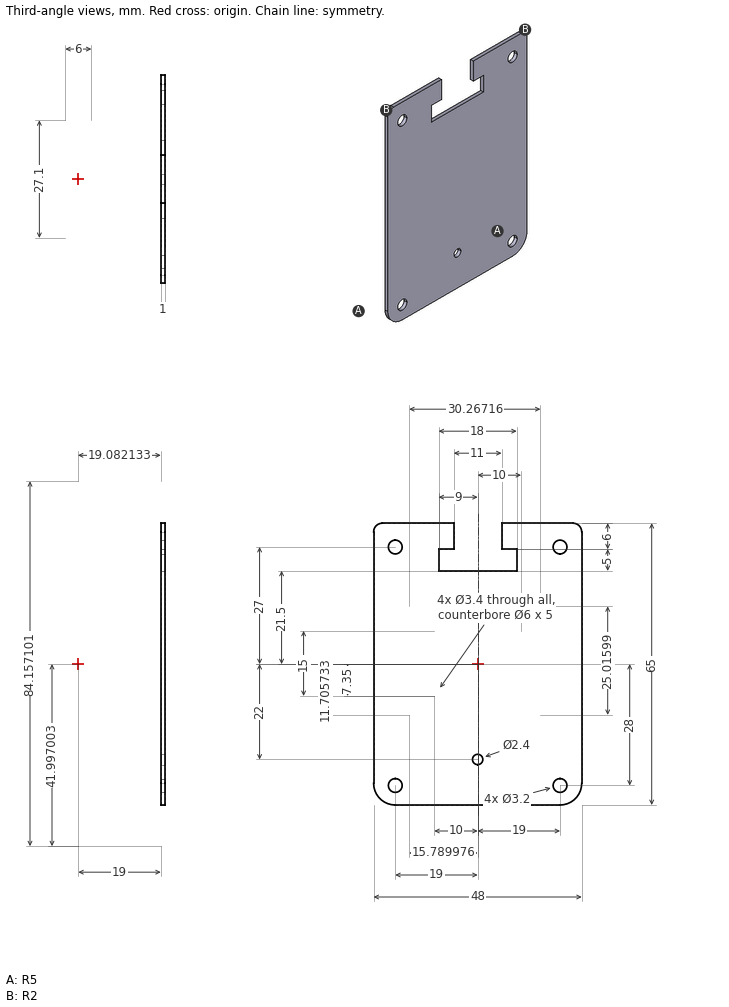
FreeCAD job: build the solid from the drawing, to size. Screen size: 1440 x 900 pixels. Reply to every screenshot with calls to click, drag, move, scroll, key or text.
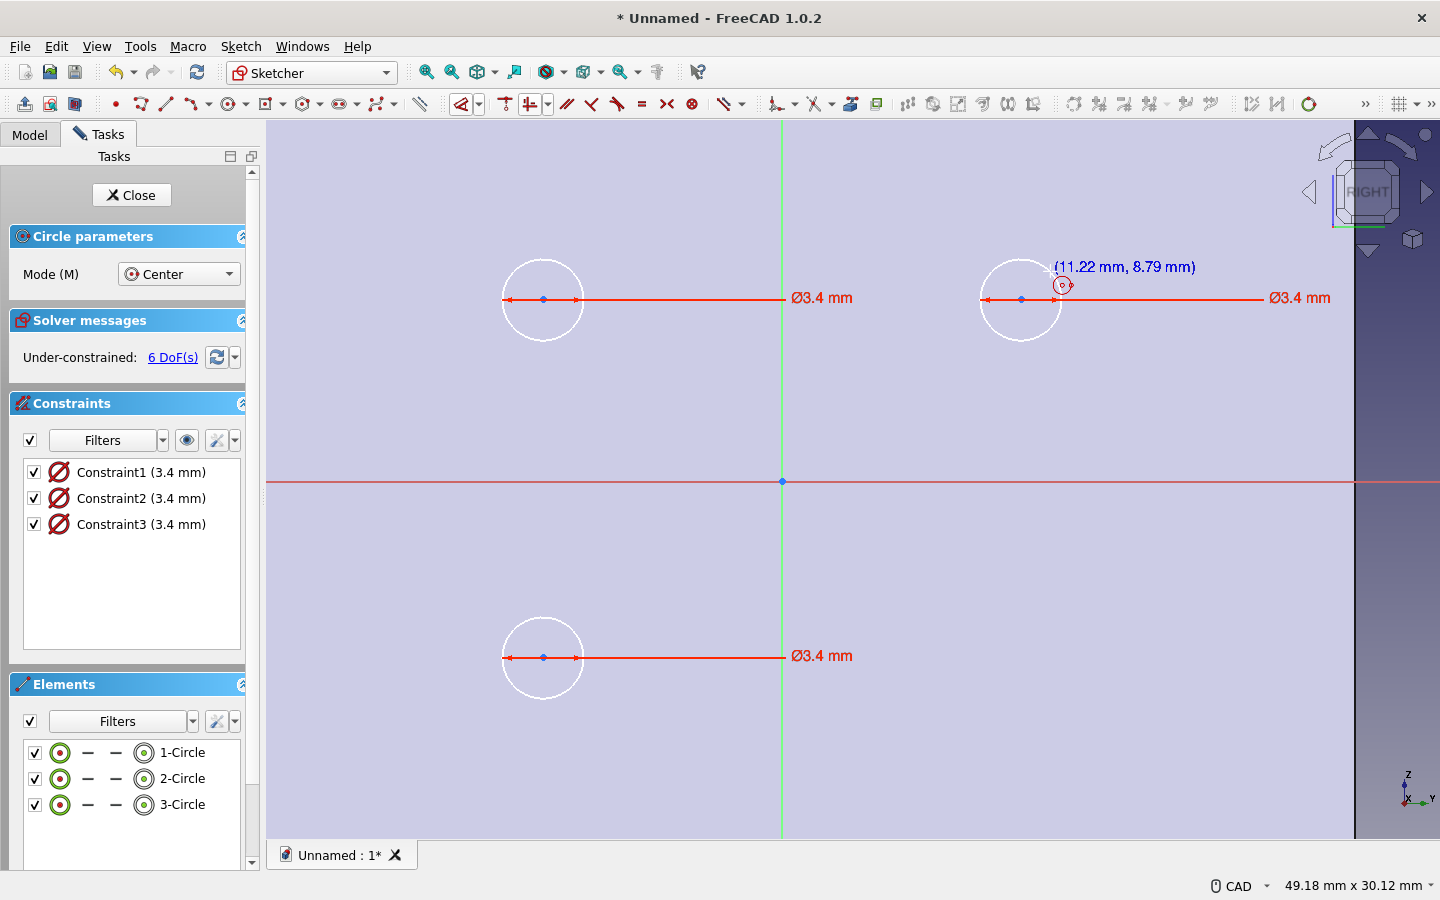
click(1021, 657)
move(1050, 629)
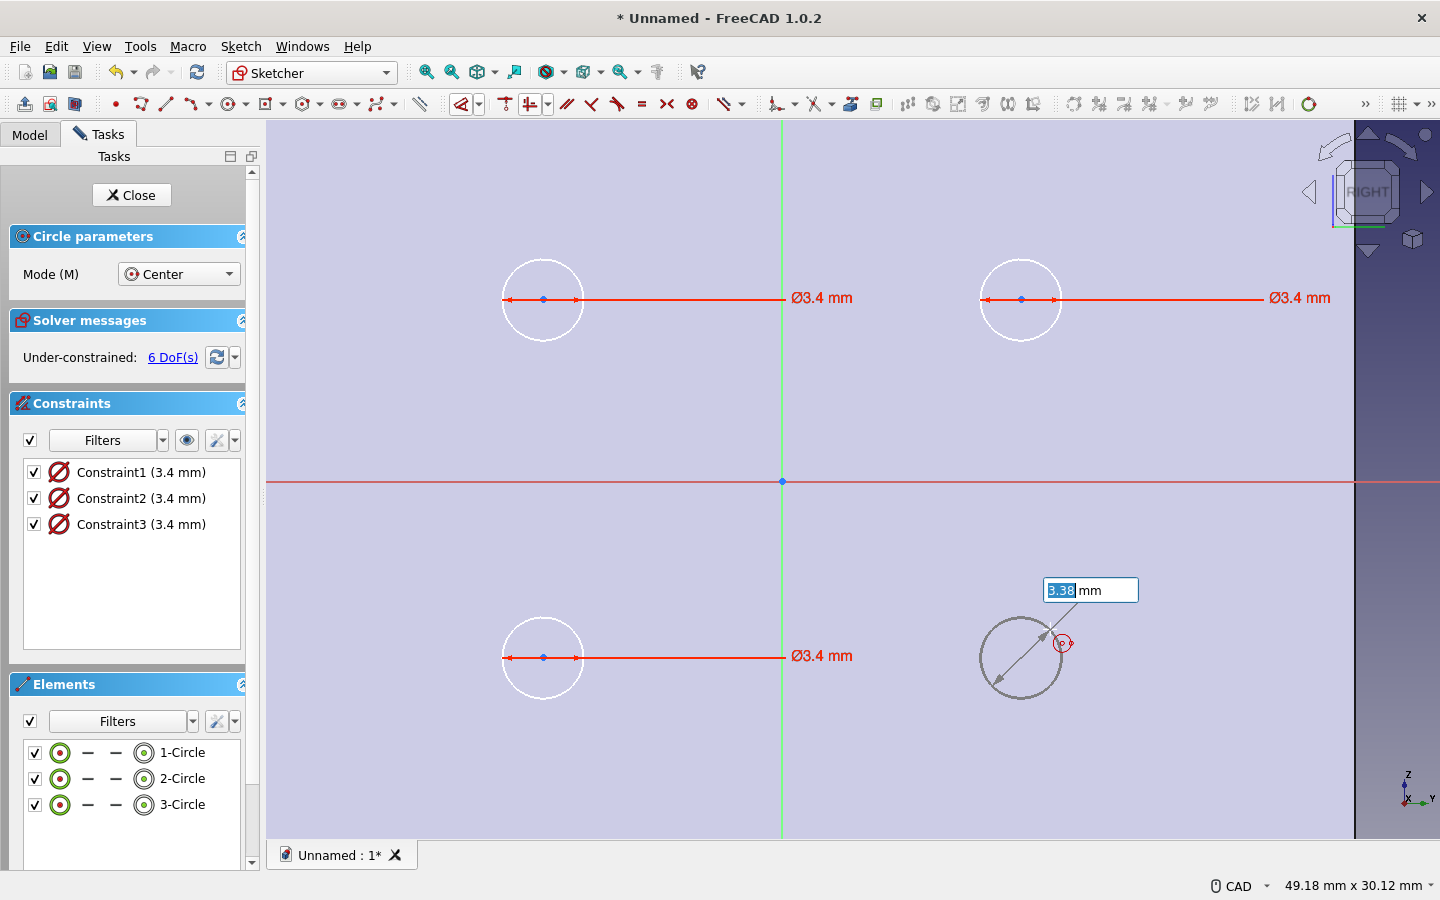
text(3.4)
key(Return)
key(Escape)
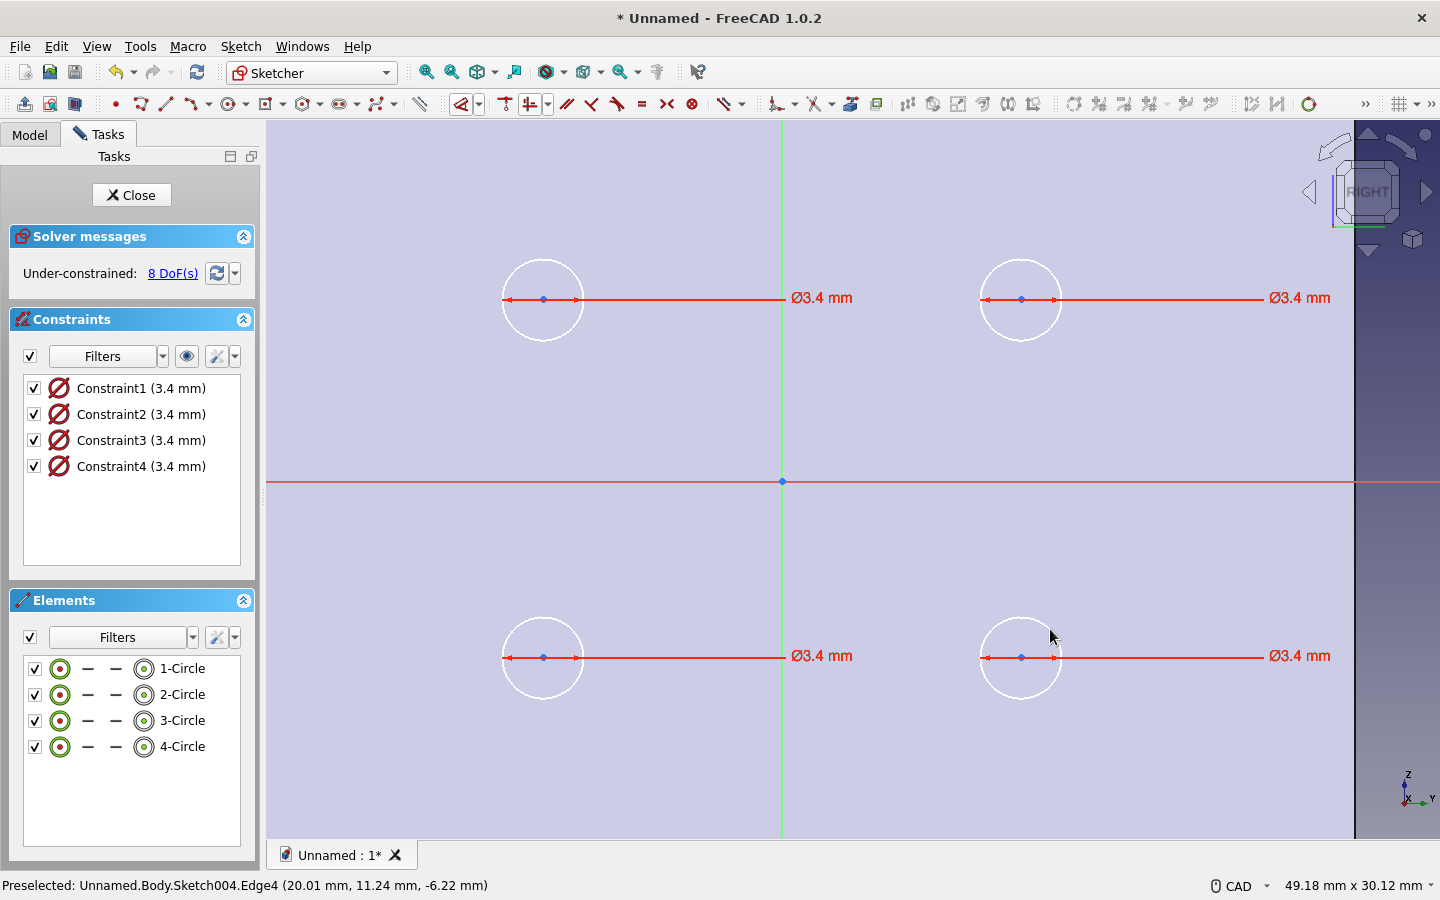
click(543, 658)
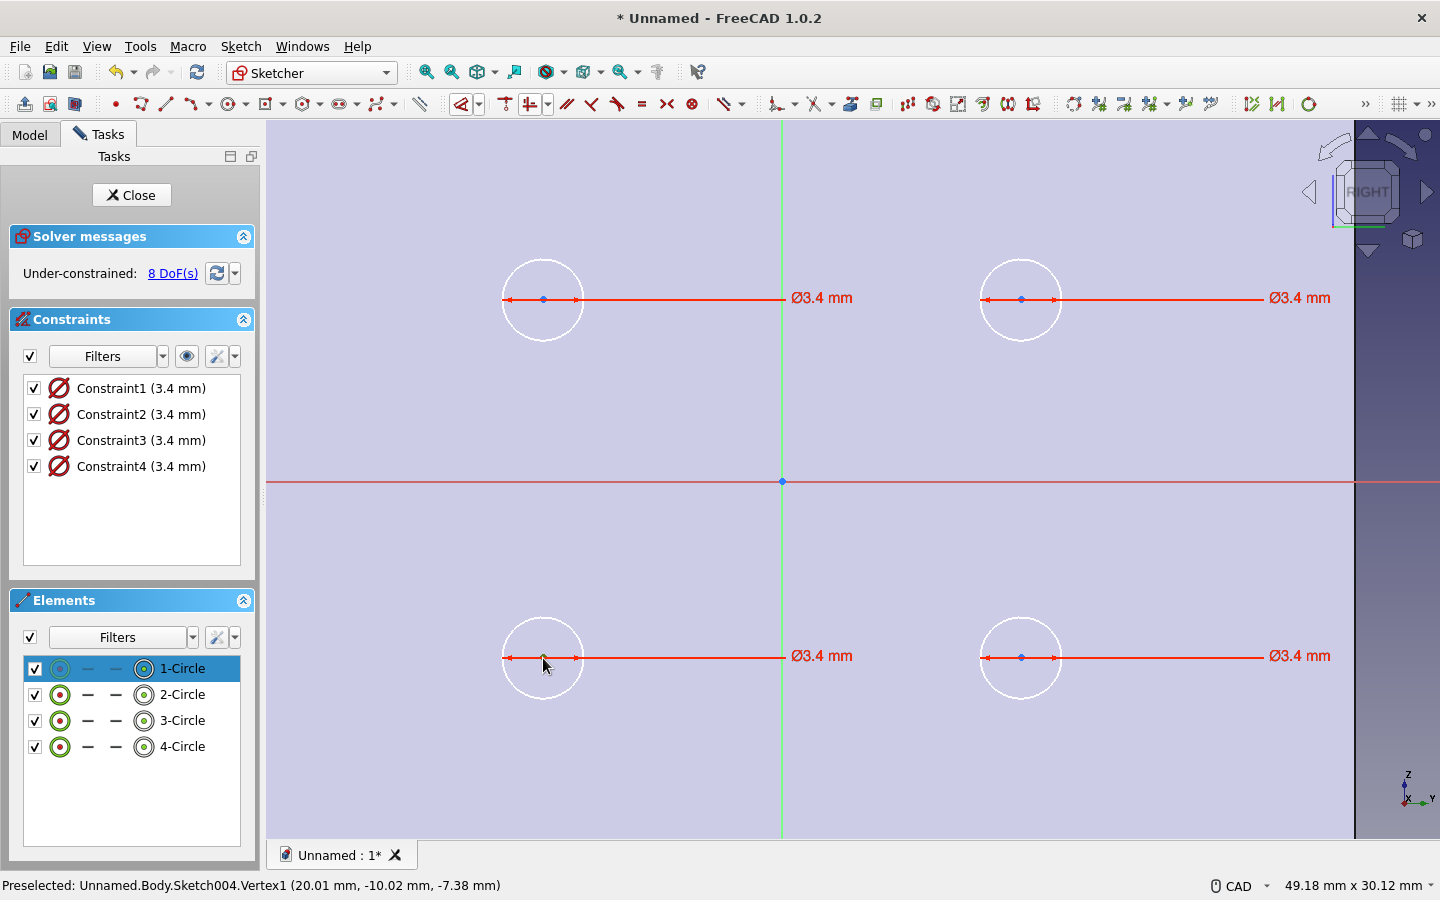
click(543, 300)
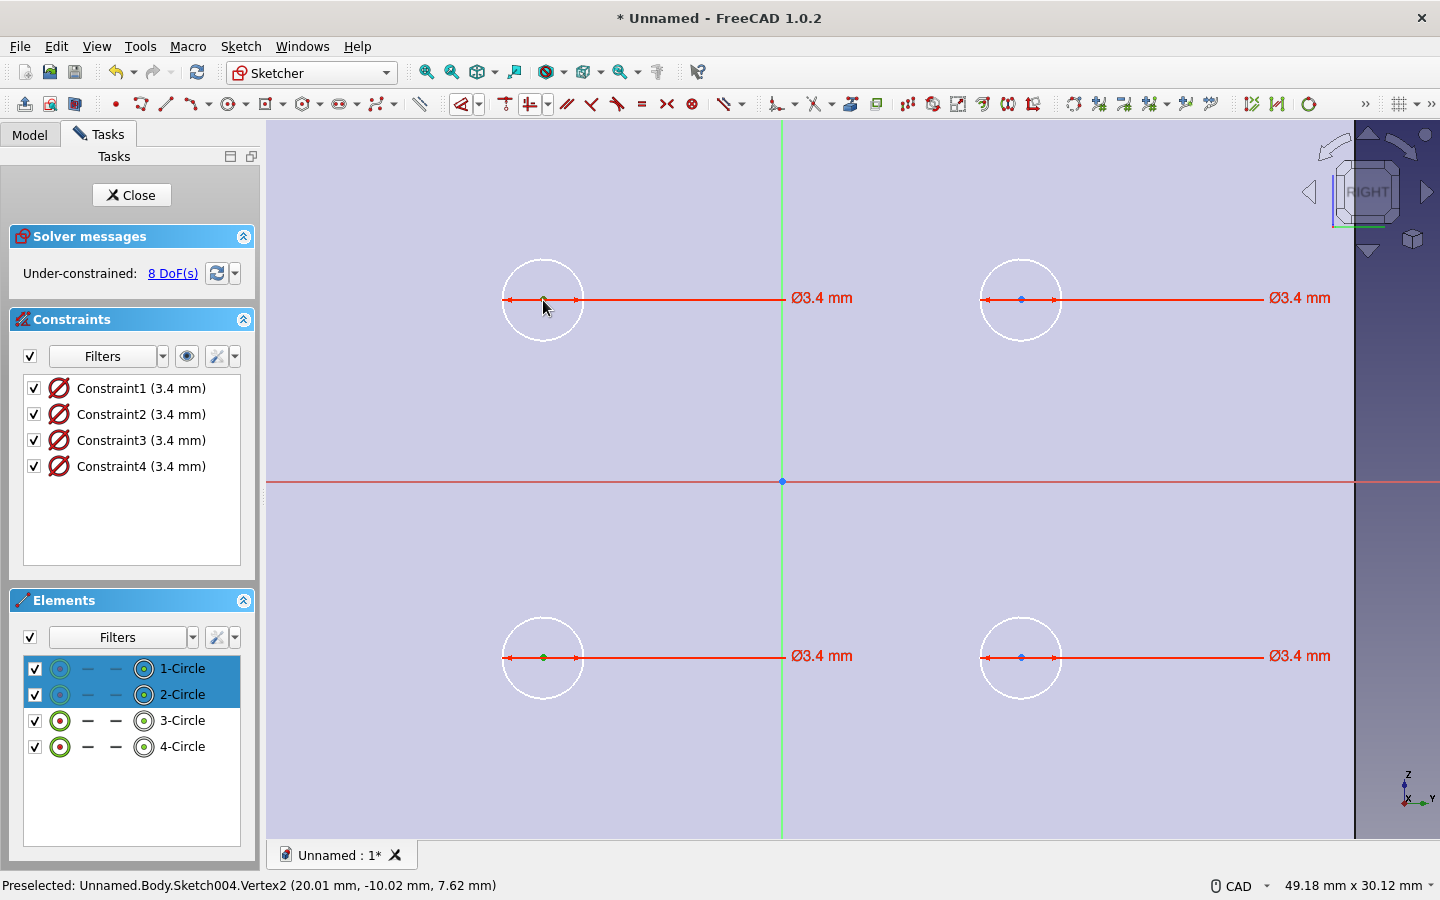
key(v)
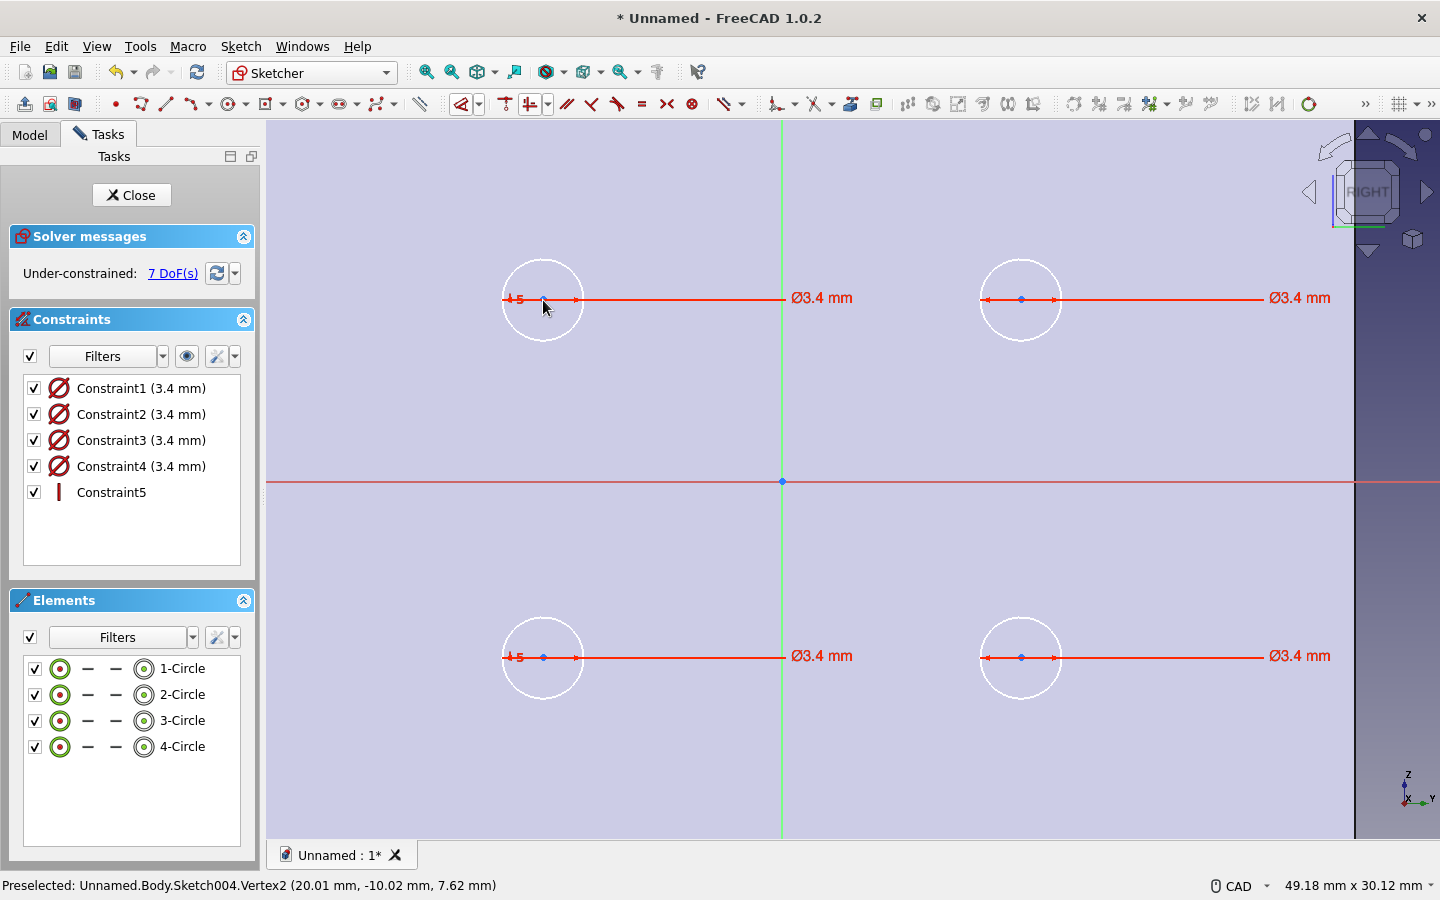
click(543, 300)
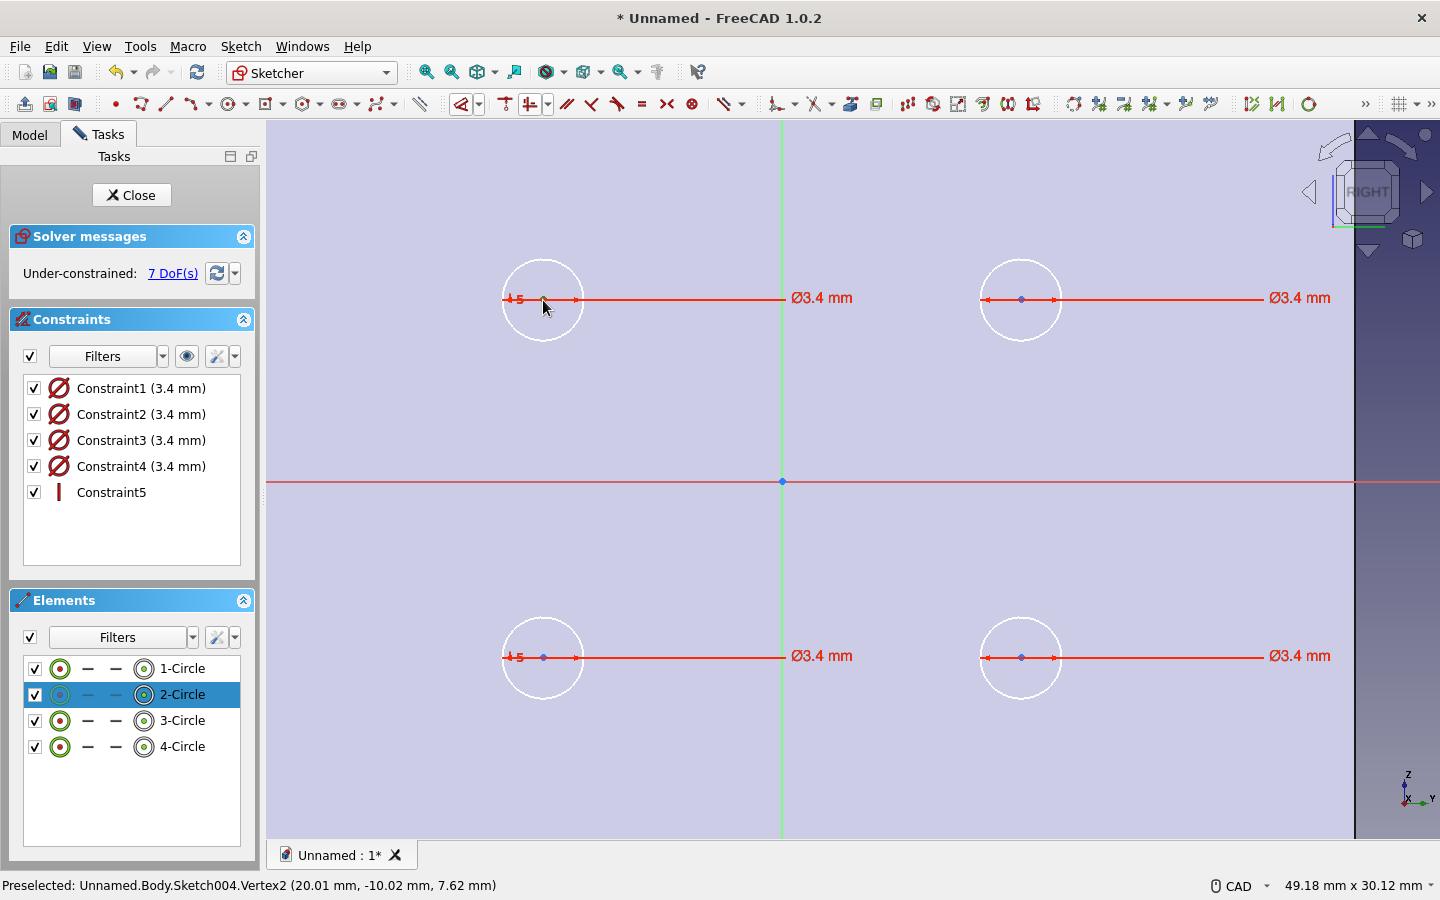
click(1021, 300)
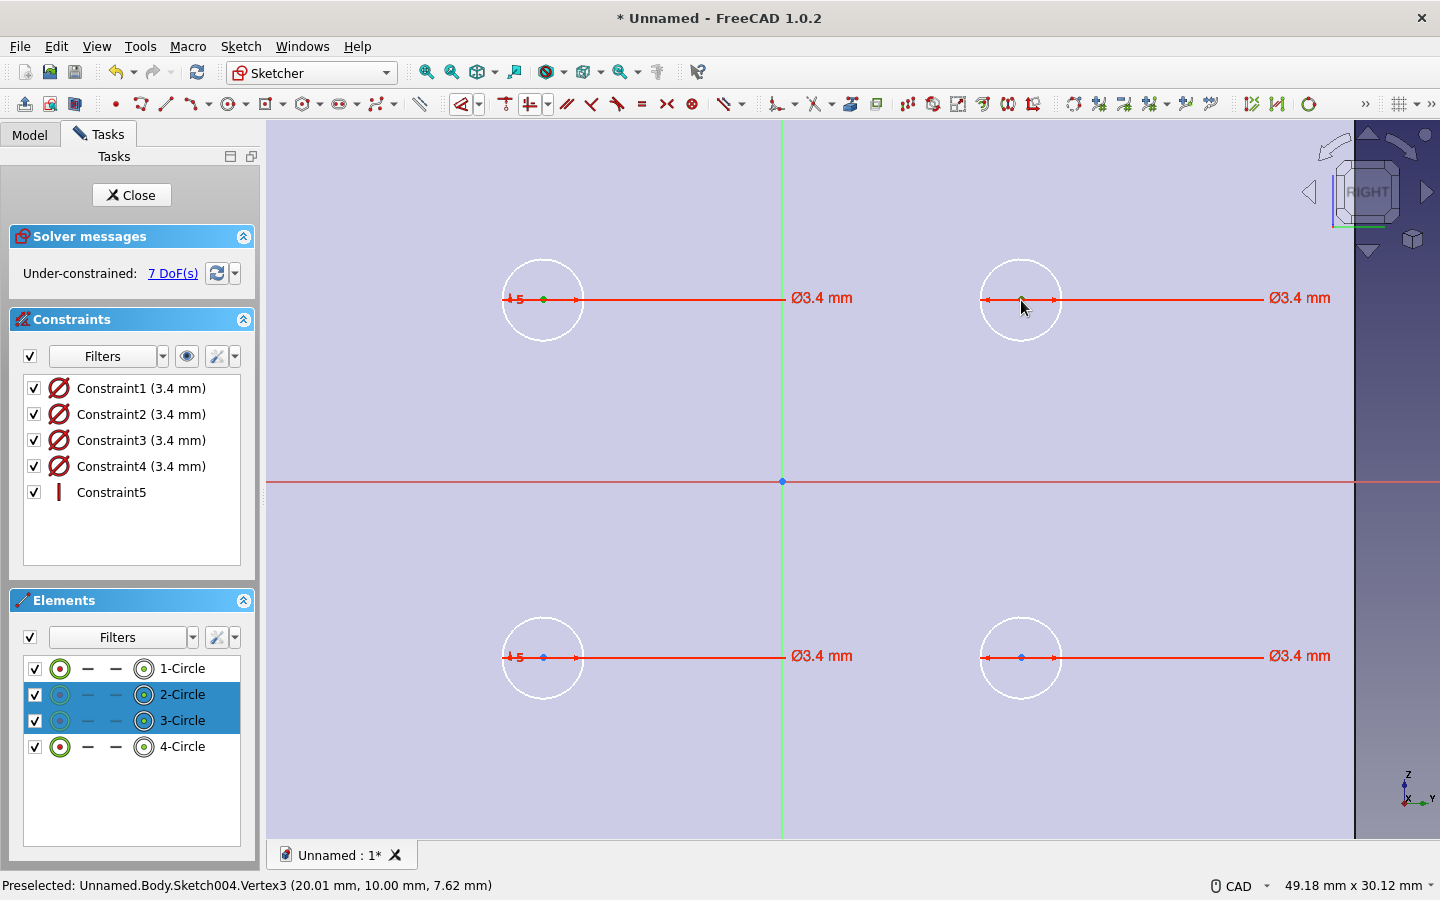
key(h)